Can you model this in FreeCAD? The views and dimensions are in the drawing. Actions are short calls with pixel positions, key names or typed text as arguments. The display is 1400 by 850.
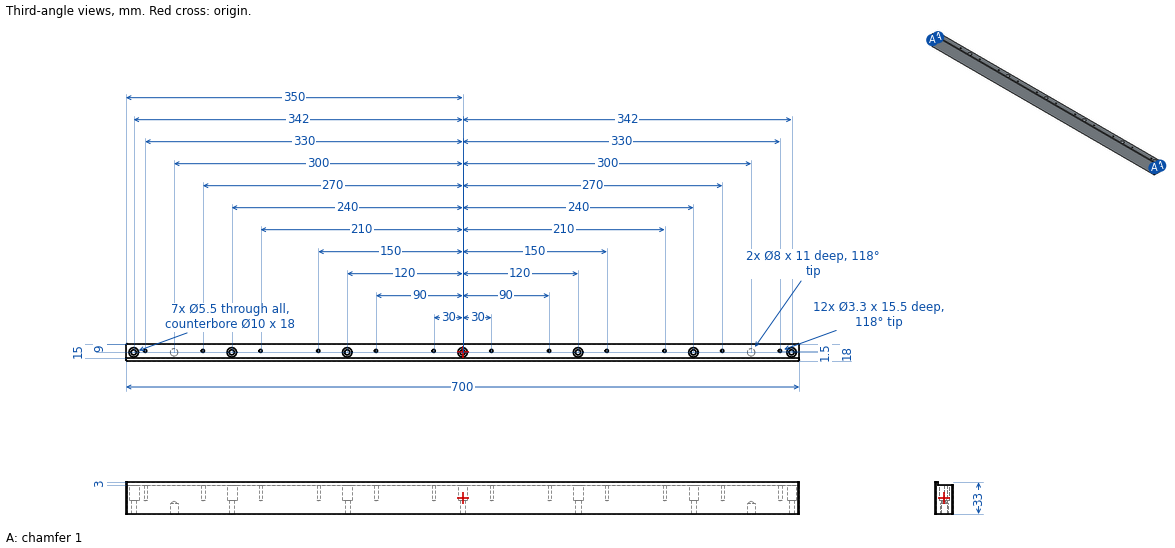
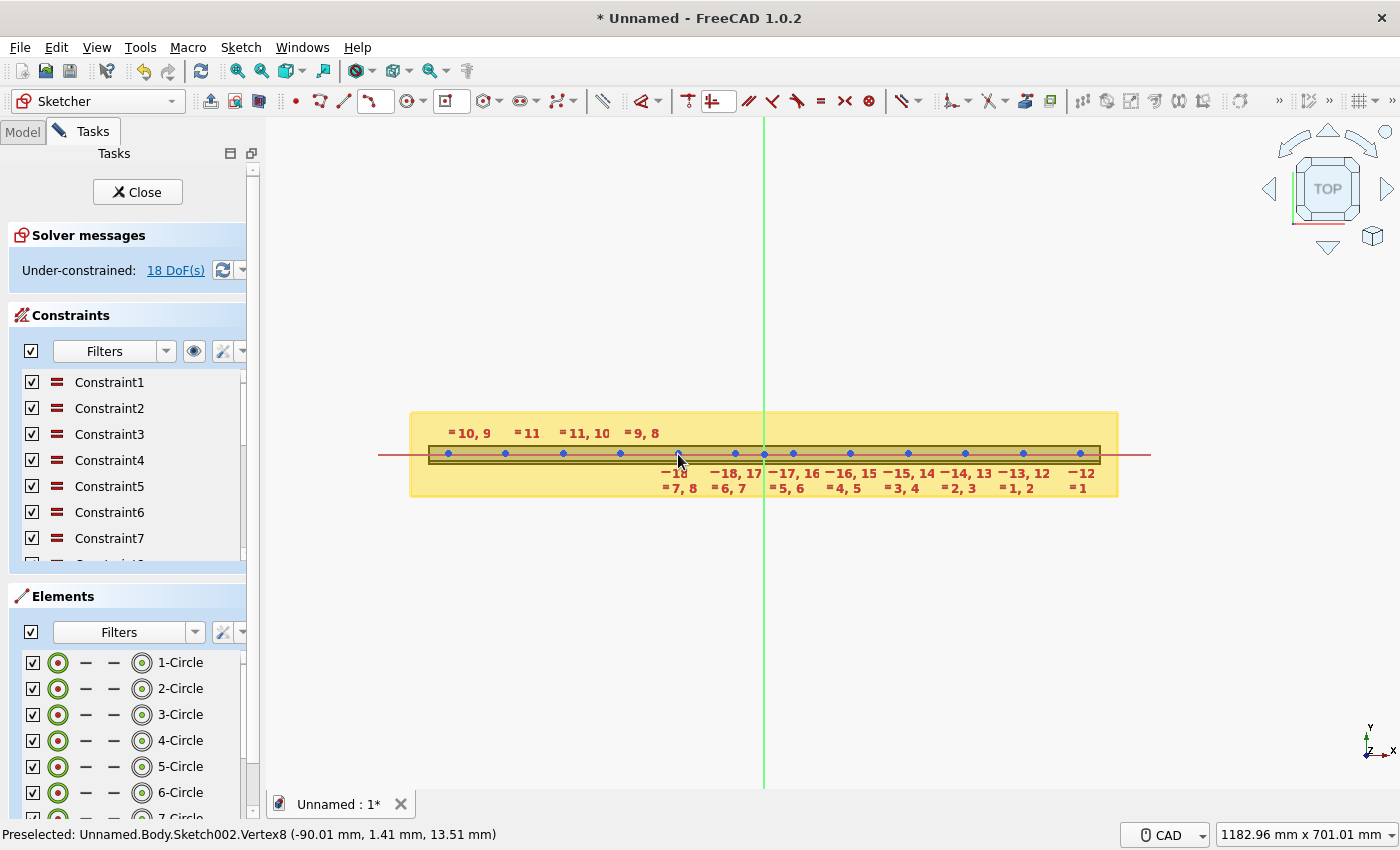
click(678, 453)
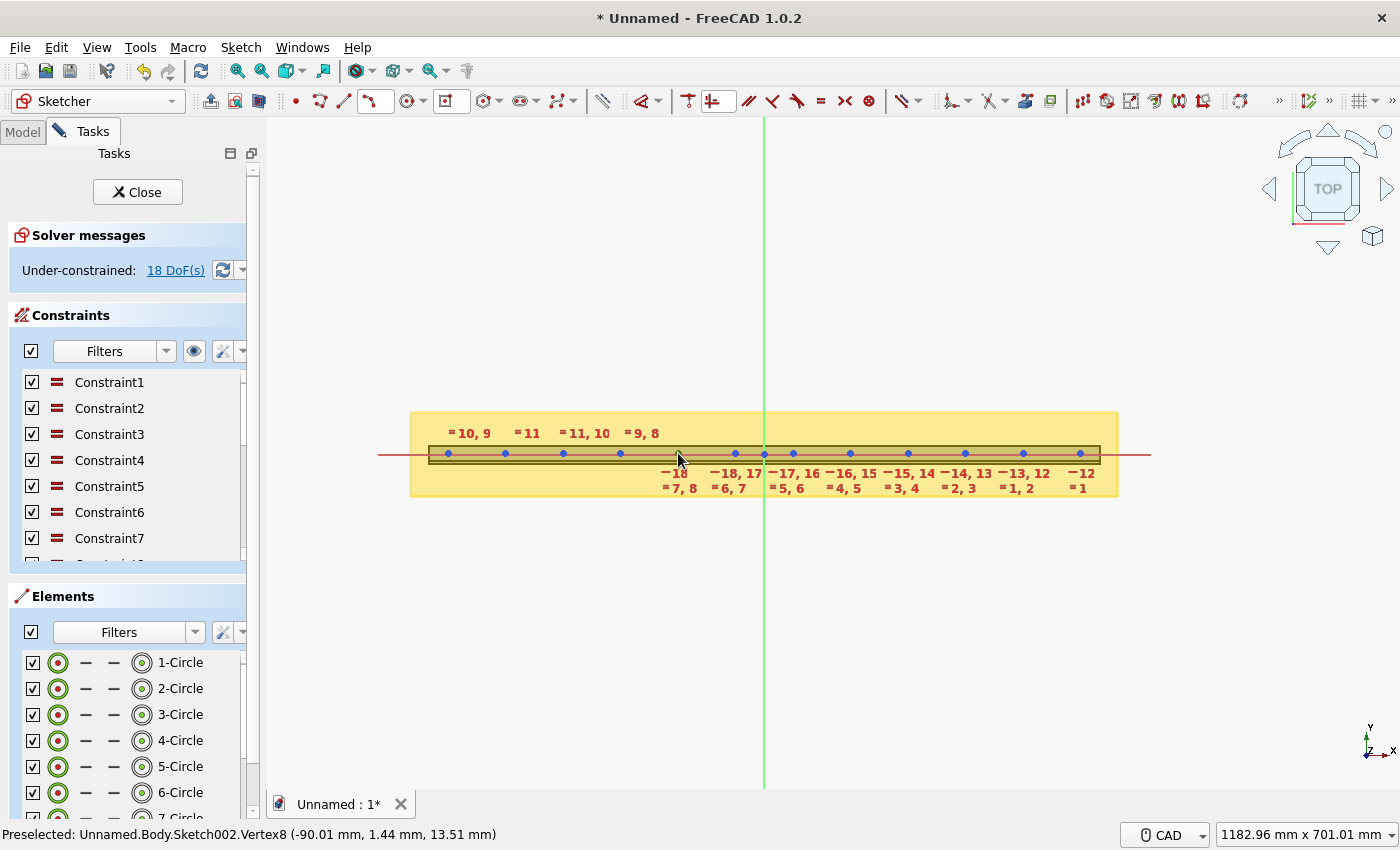
click(621, 454)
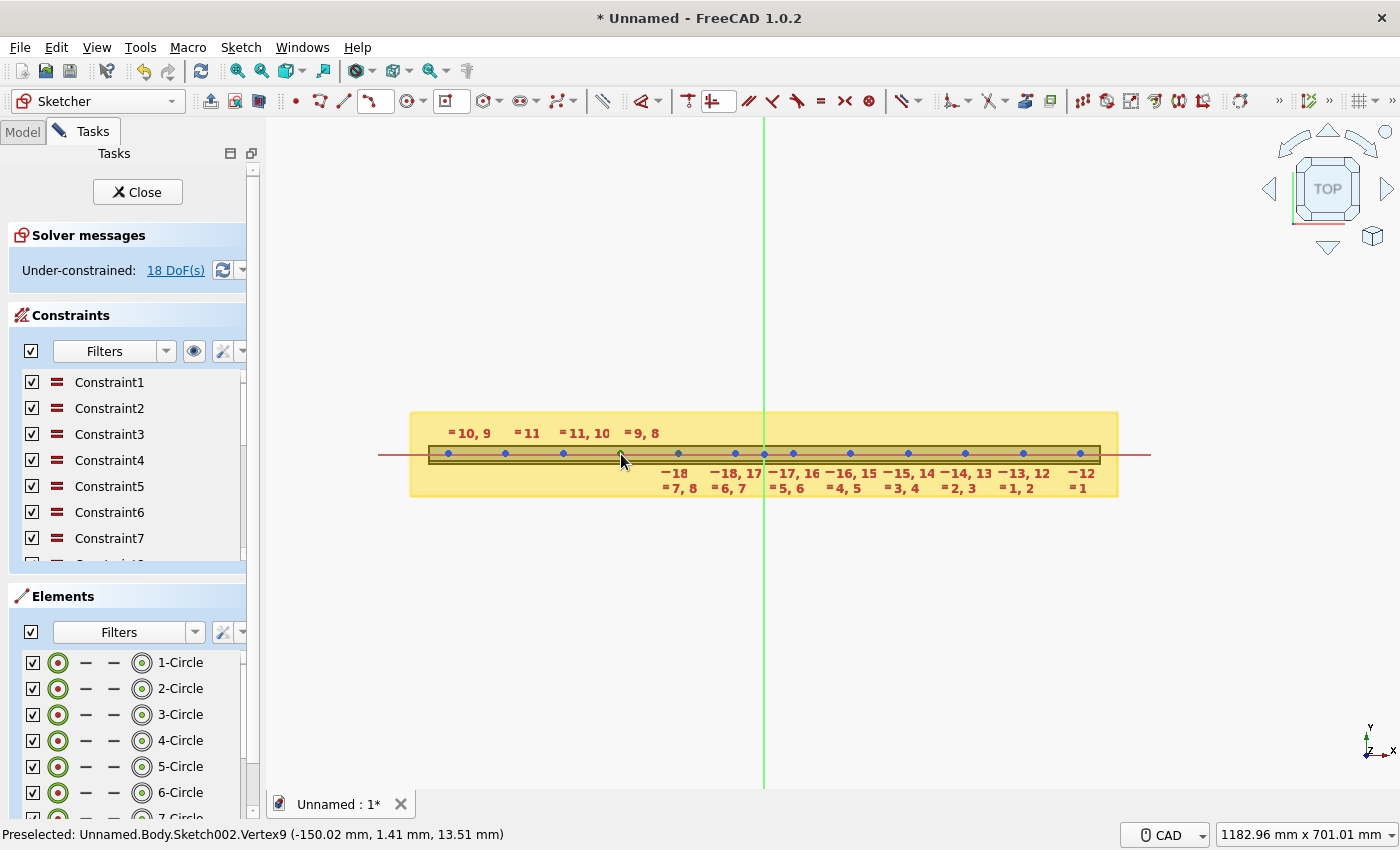
key(h)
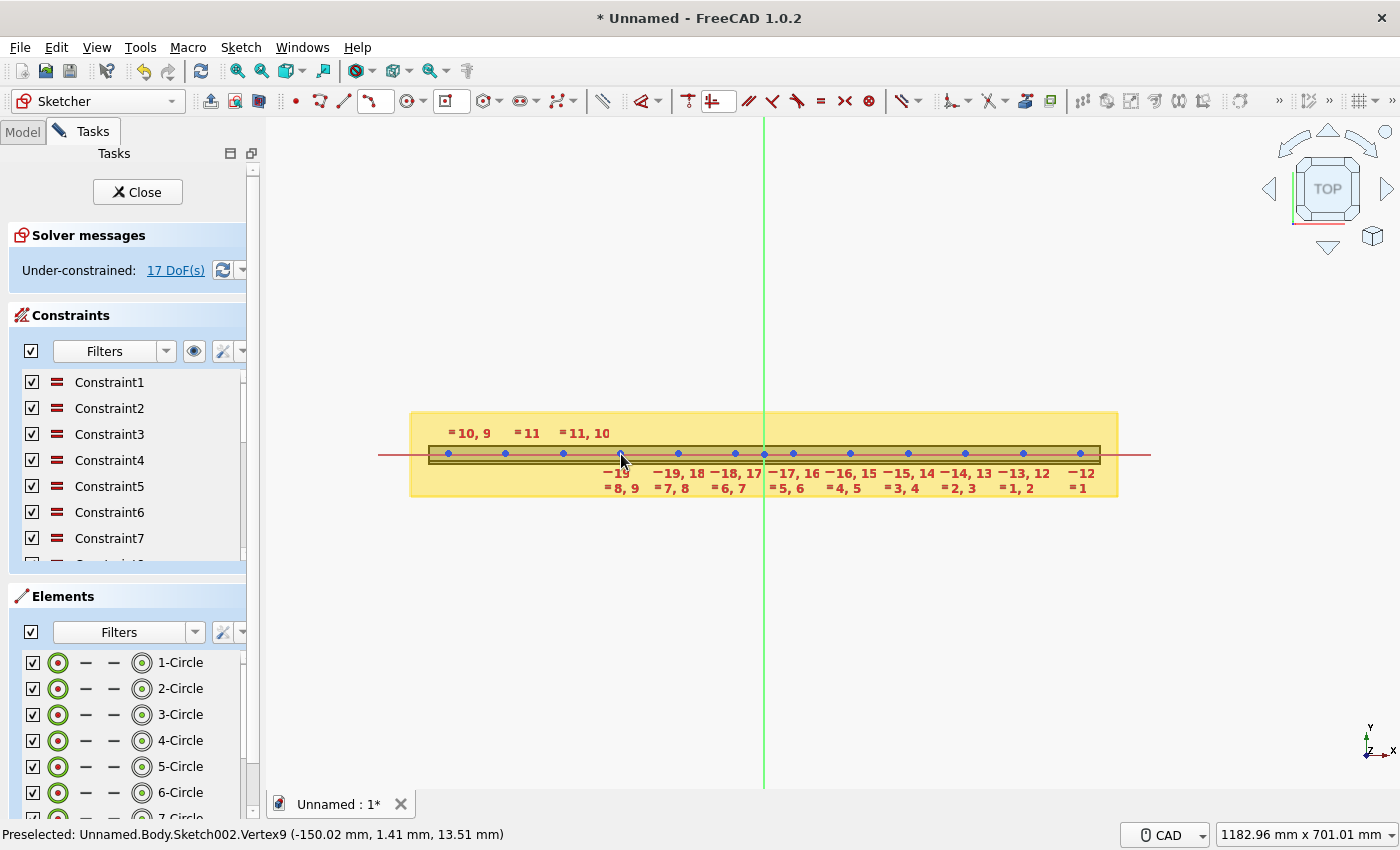
click(621, 453)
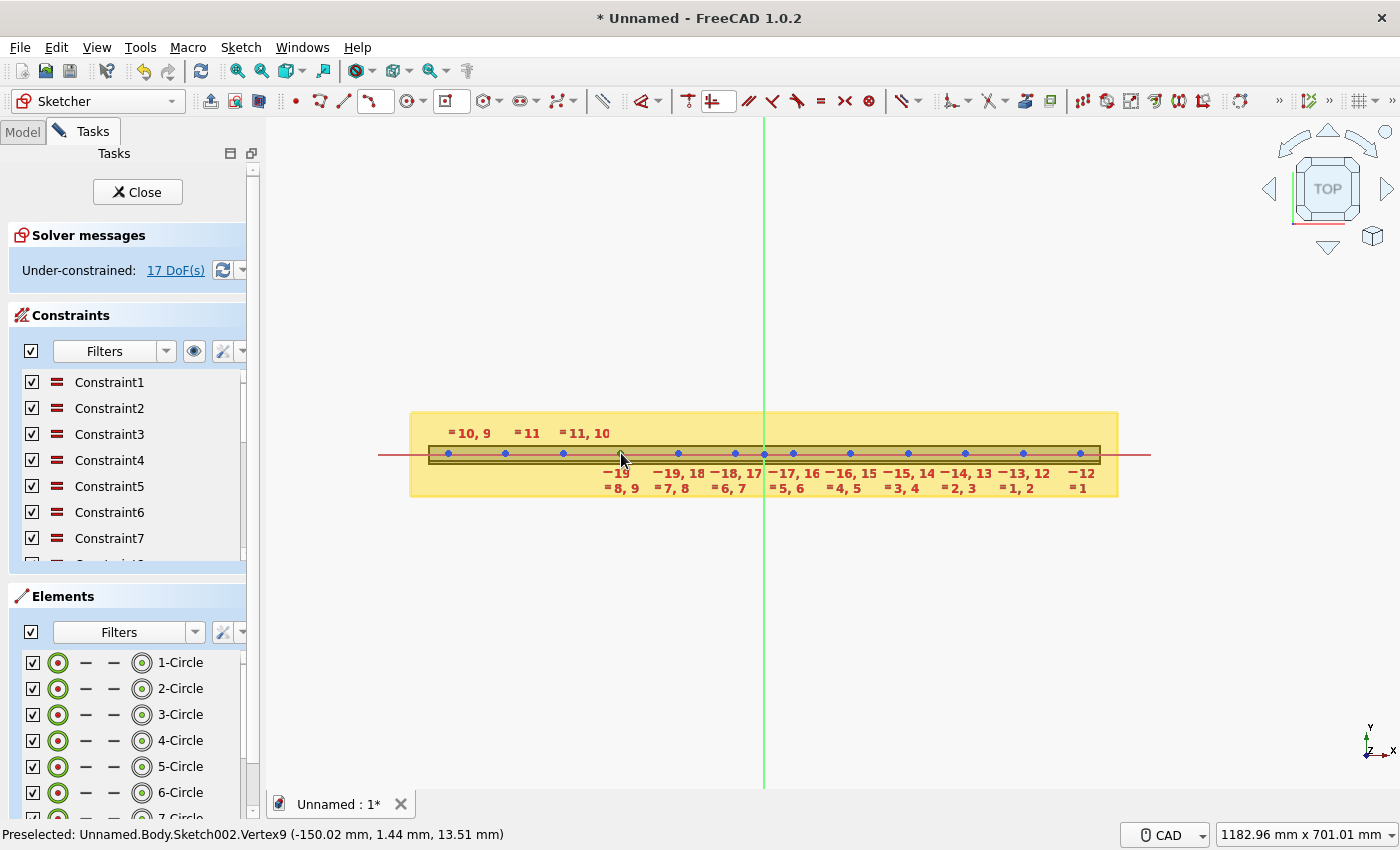
click(448, 454)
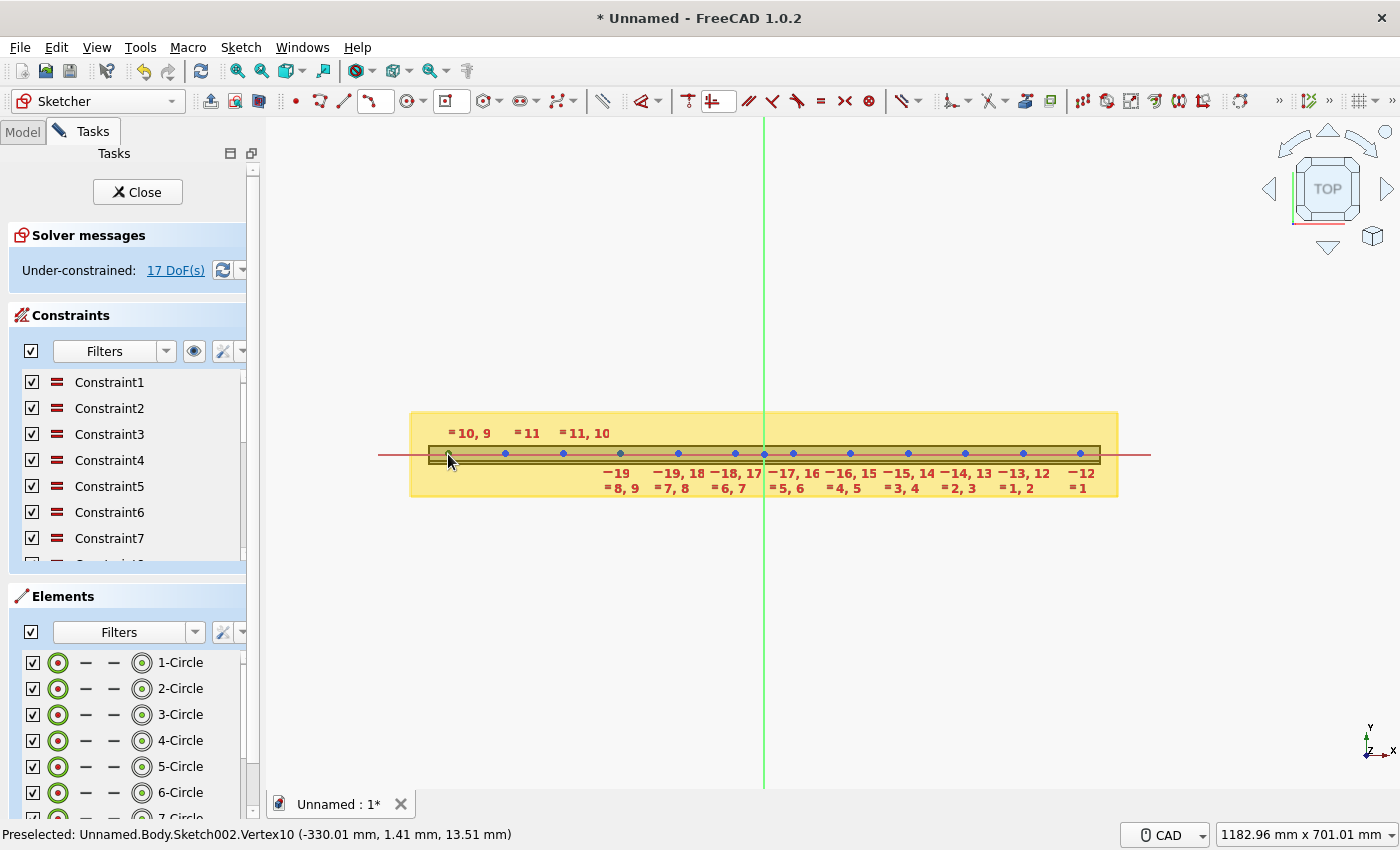
key(h)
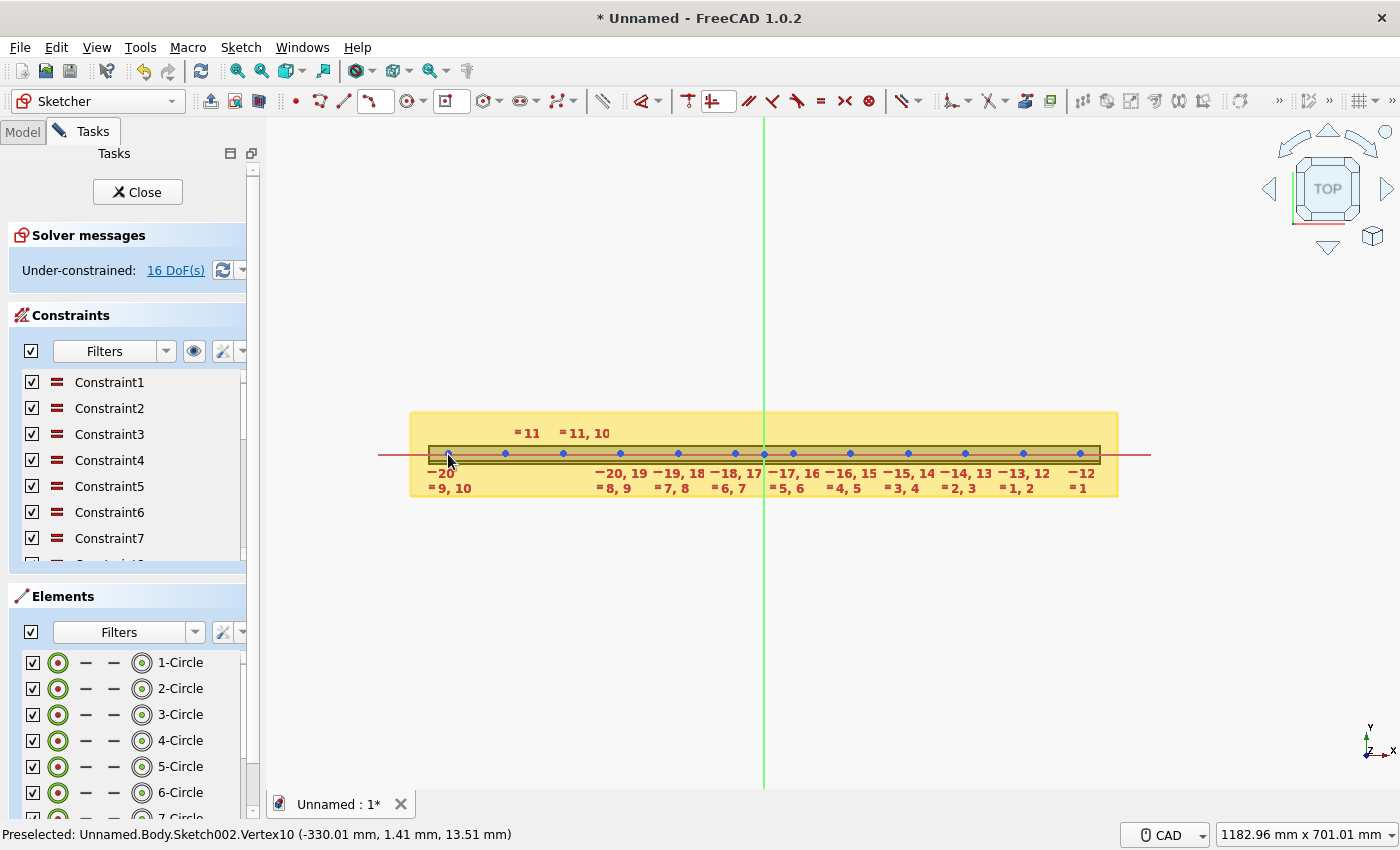
click(621, 453)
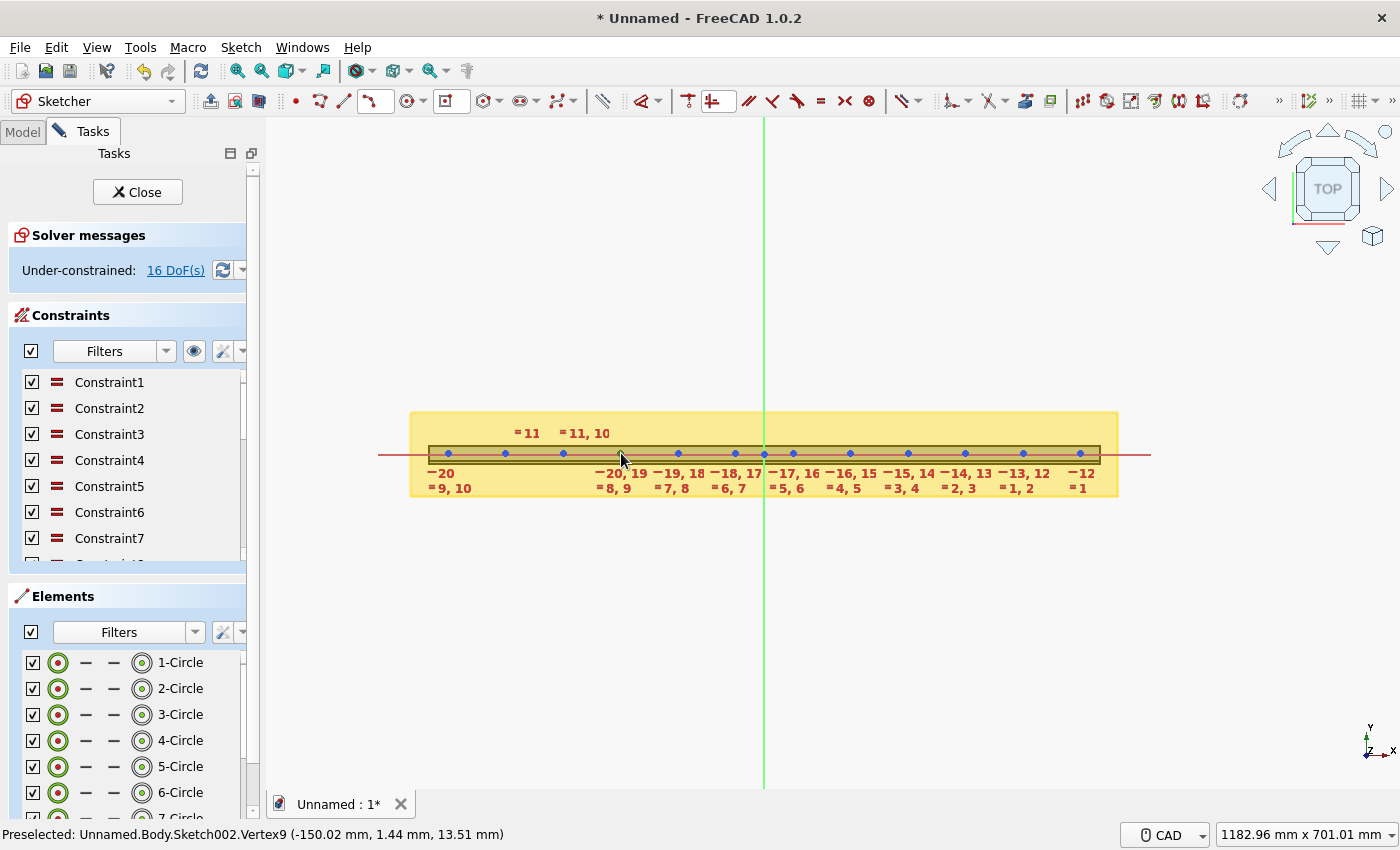
click(563, 454)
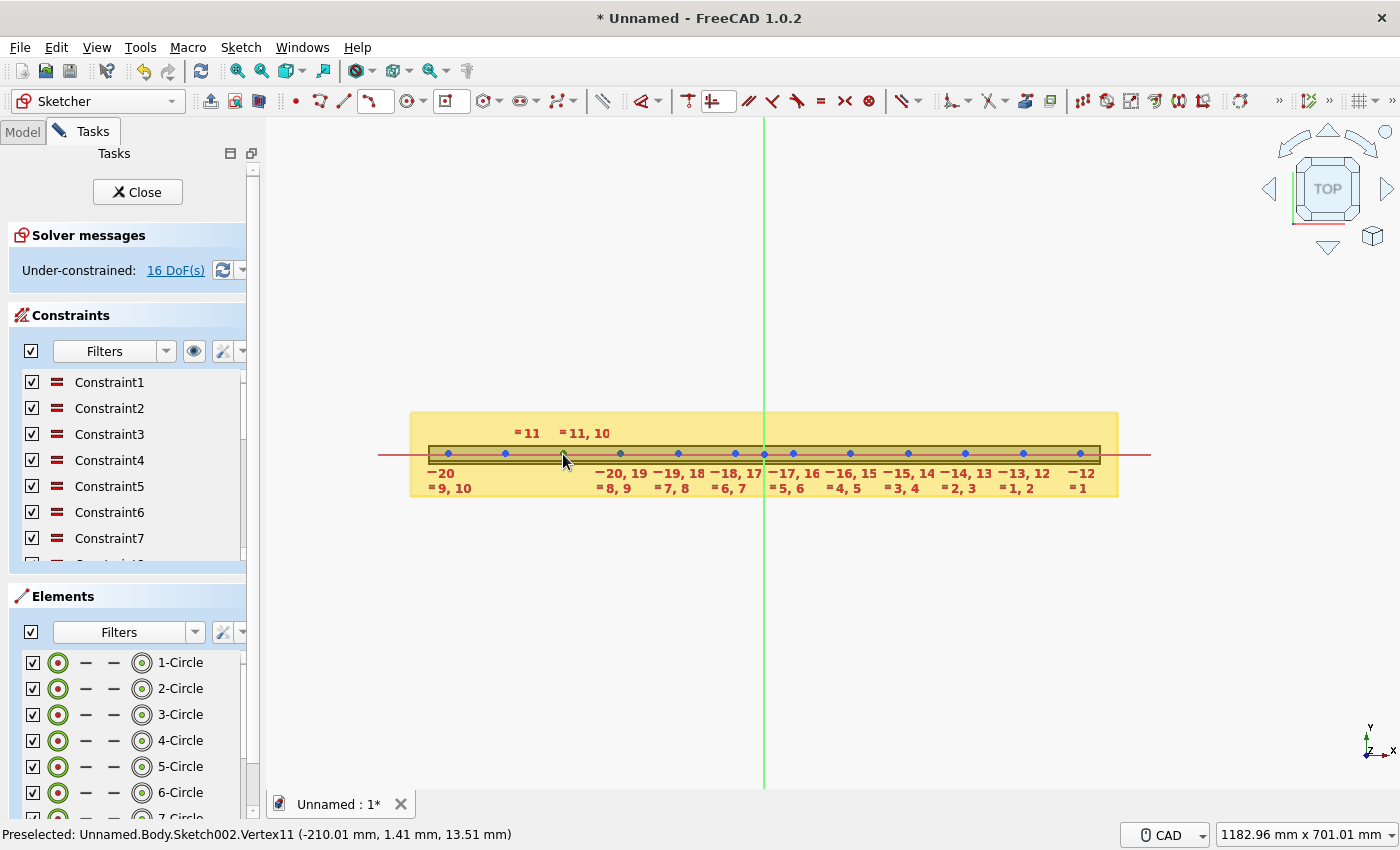
key(h)